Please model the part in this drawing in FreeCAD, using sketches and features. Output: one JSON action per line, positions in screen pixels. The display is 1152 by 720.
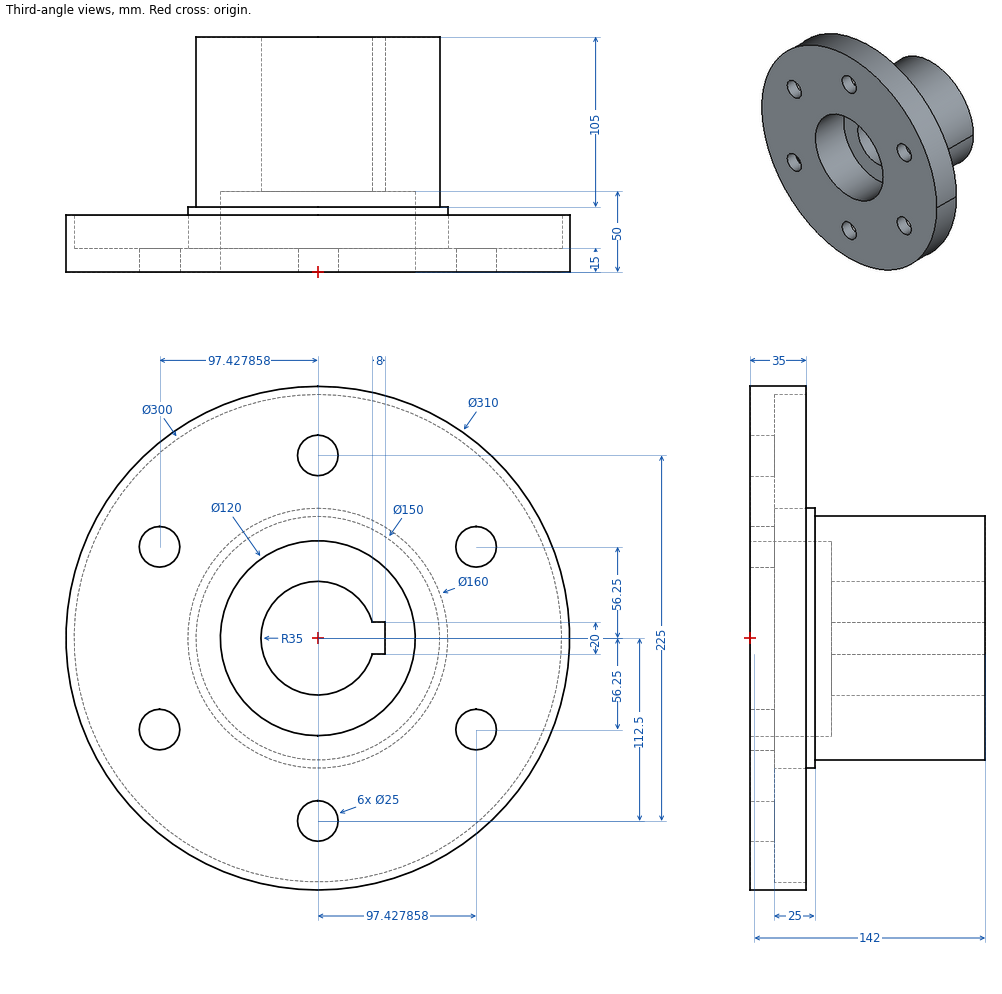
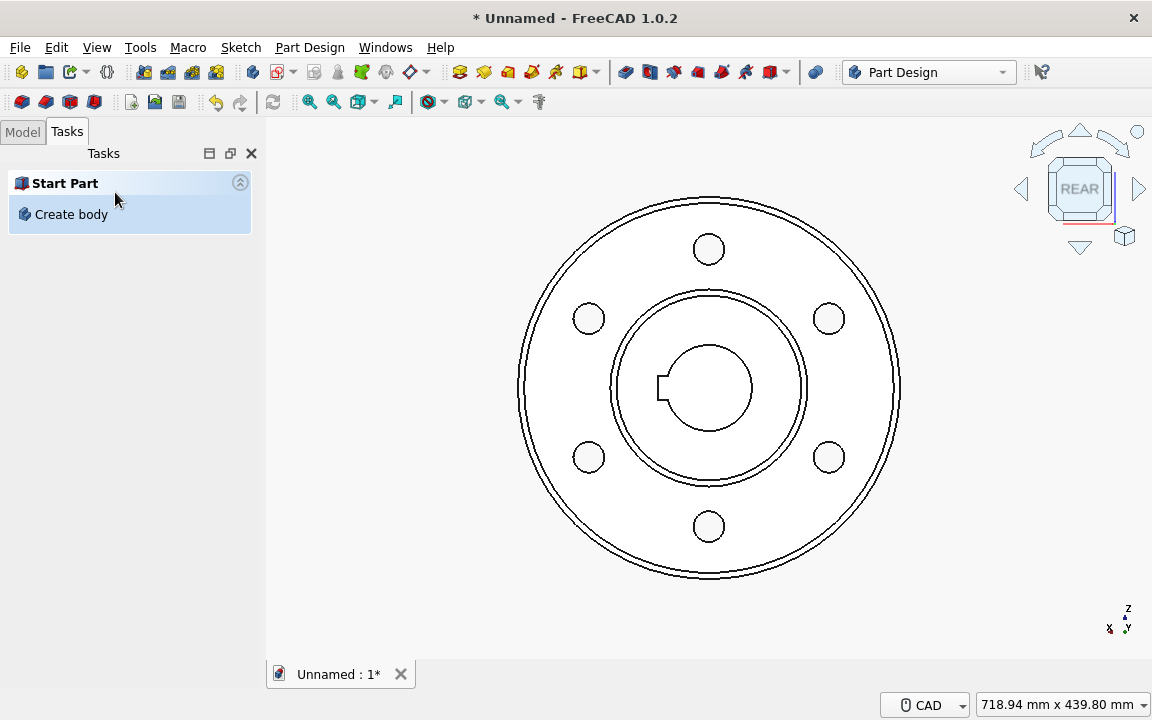
{"action": "key", "text": "0"}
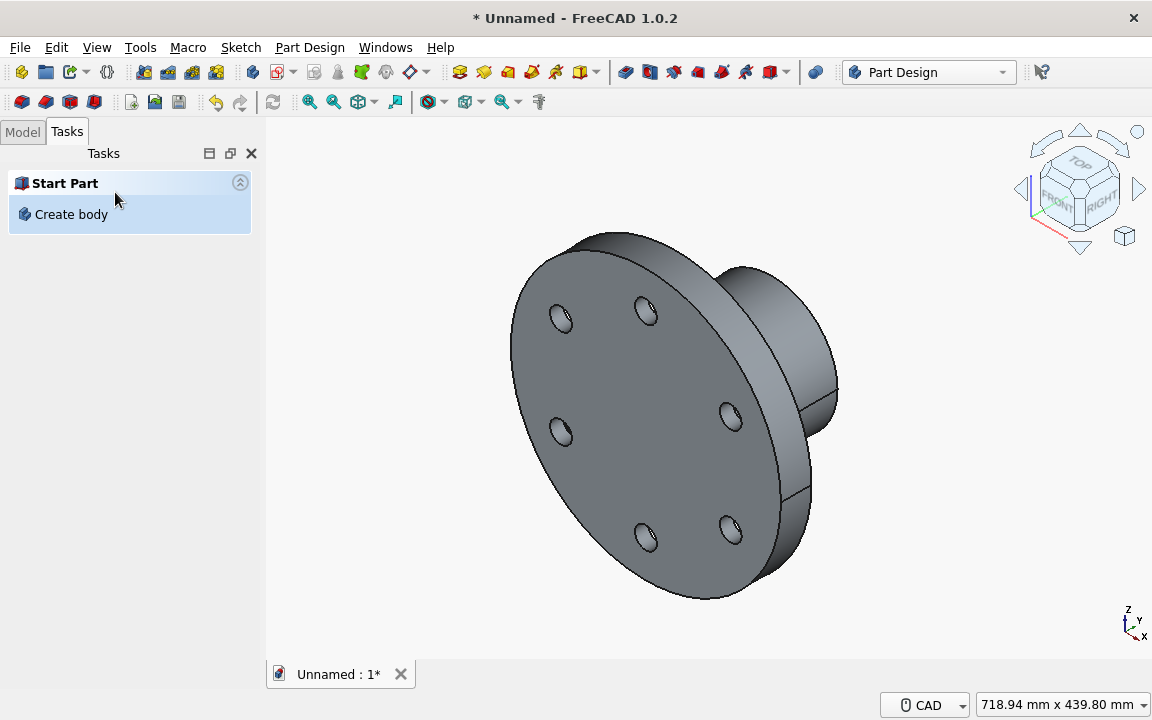
{"action": "left_click", "coordinate": [646, 423]}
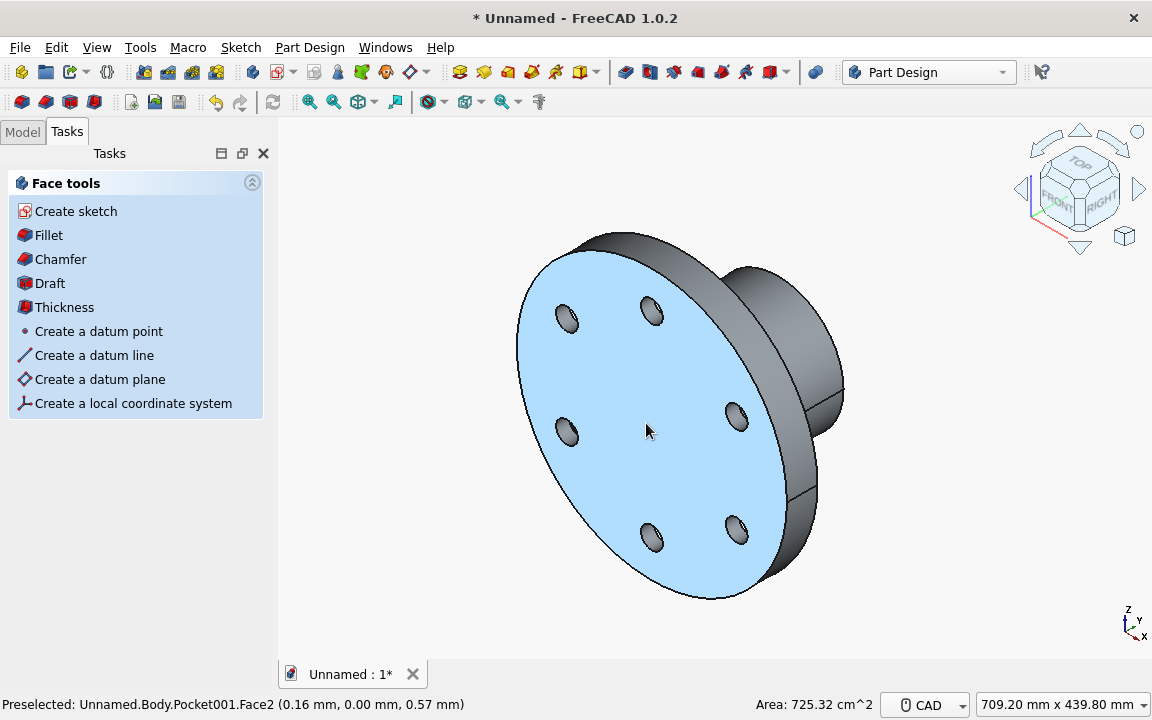
{"action": "left_click", "coordinate": [278, 72]}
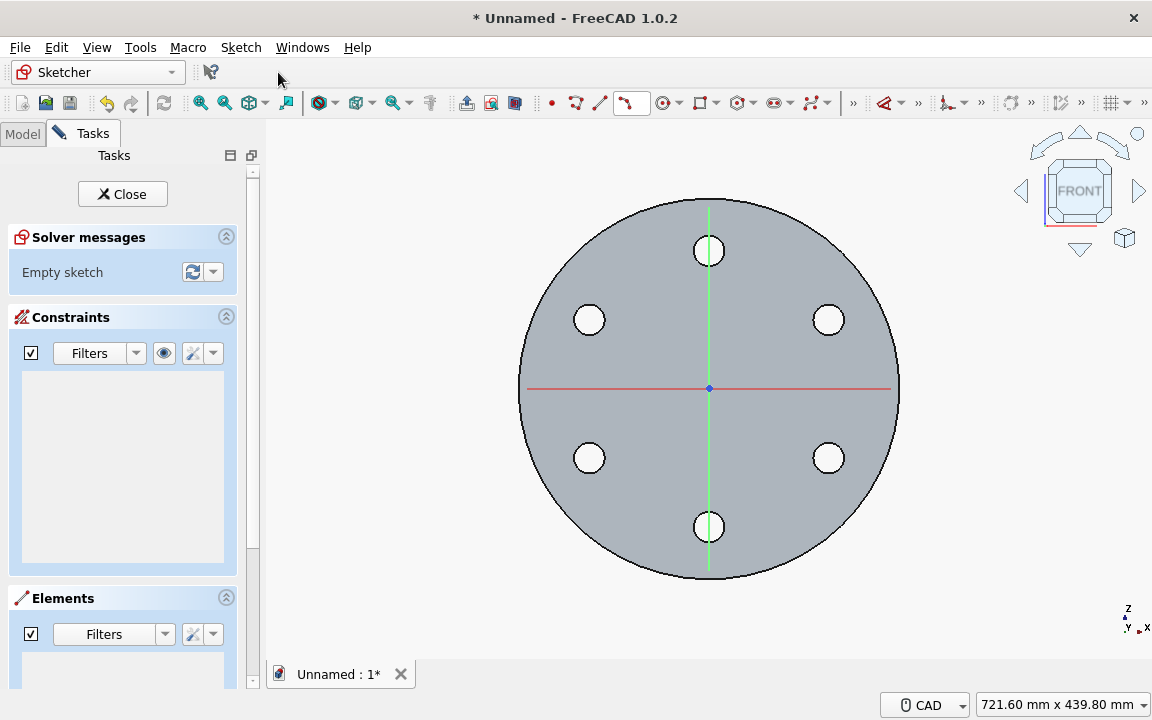
{"action": "scroll", "coordinate": [765, 389], "scroll_direction": "up", "scroll_amount": 4}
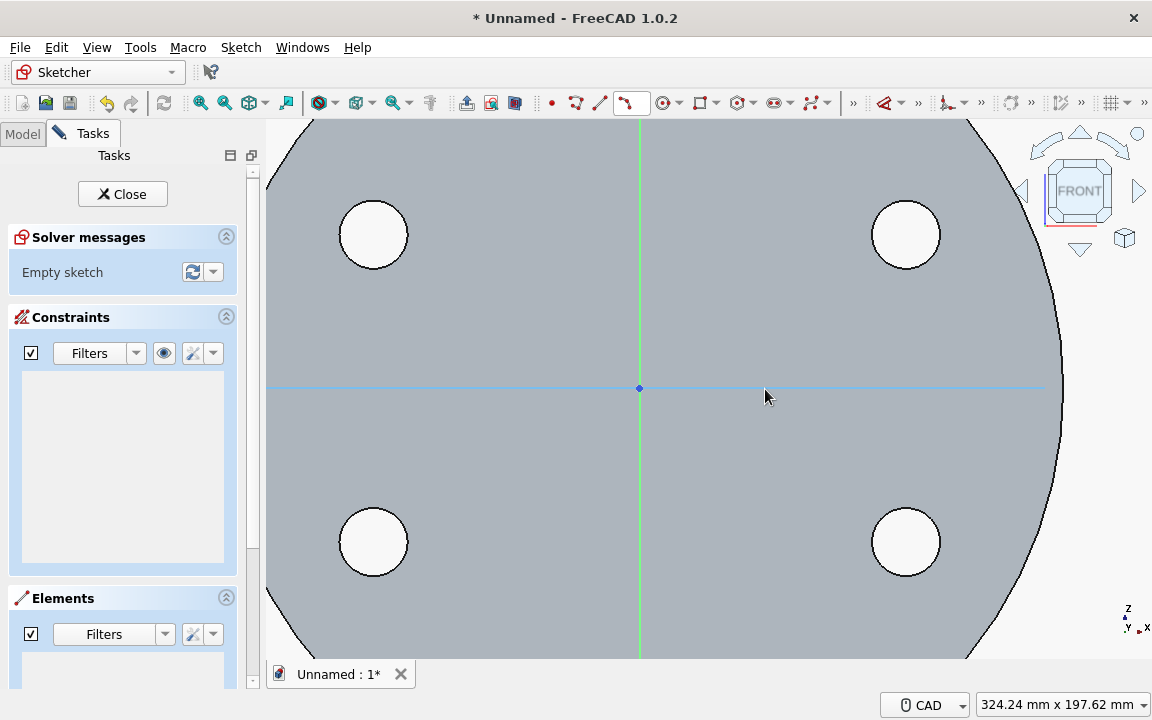
{"action": "left_click", "coordinate": [664, 104]}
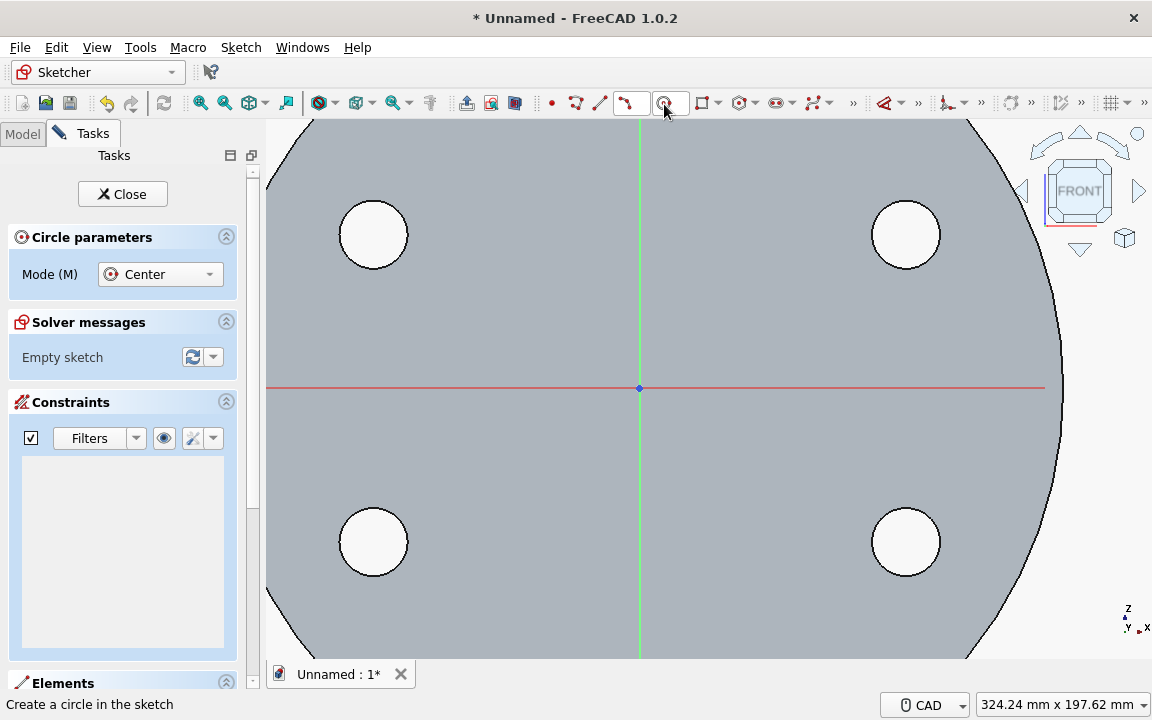
{"action": "left_click", "coordinate": [640, 388]}
{"action": "mouse_move", "coordinate": [756, 272]}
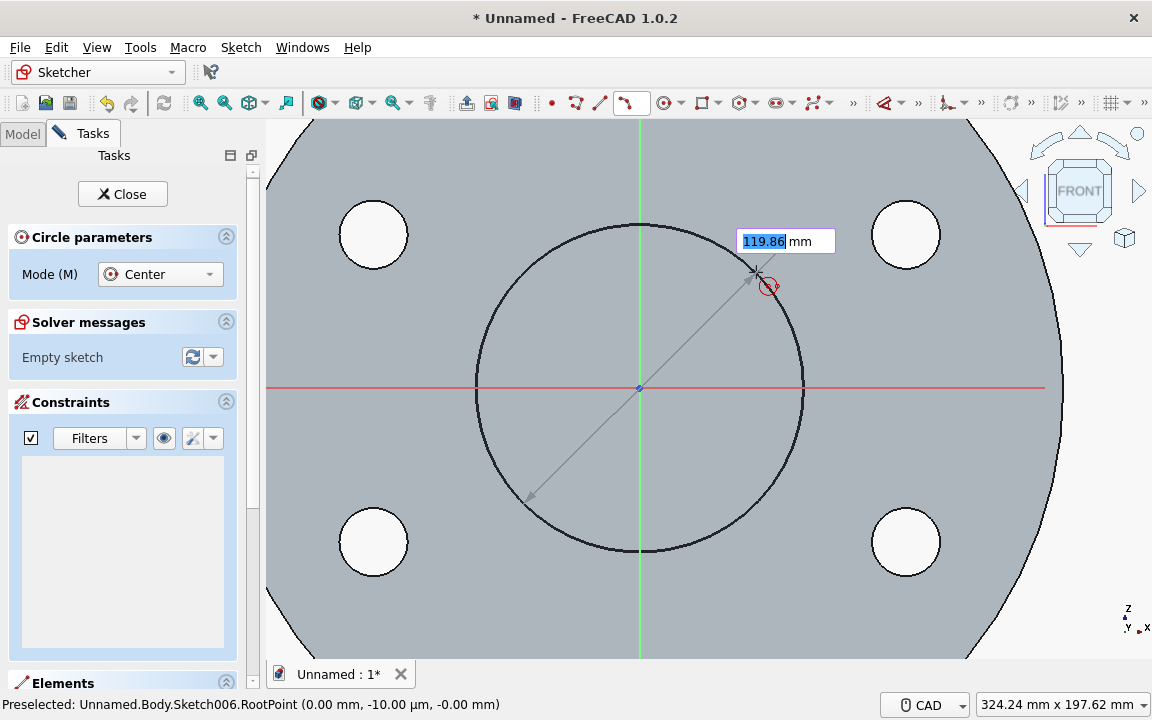
{"action": "type", "text": "120"}
{"action": "key", "text": "Return"}
{"action": "key", "text": "Escape"}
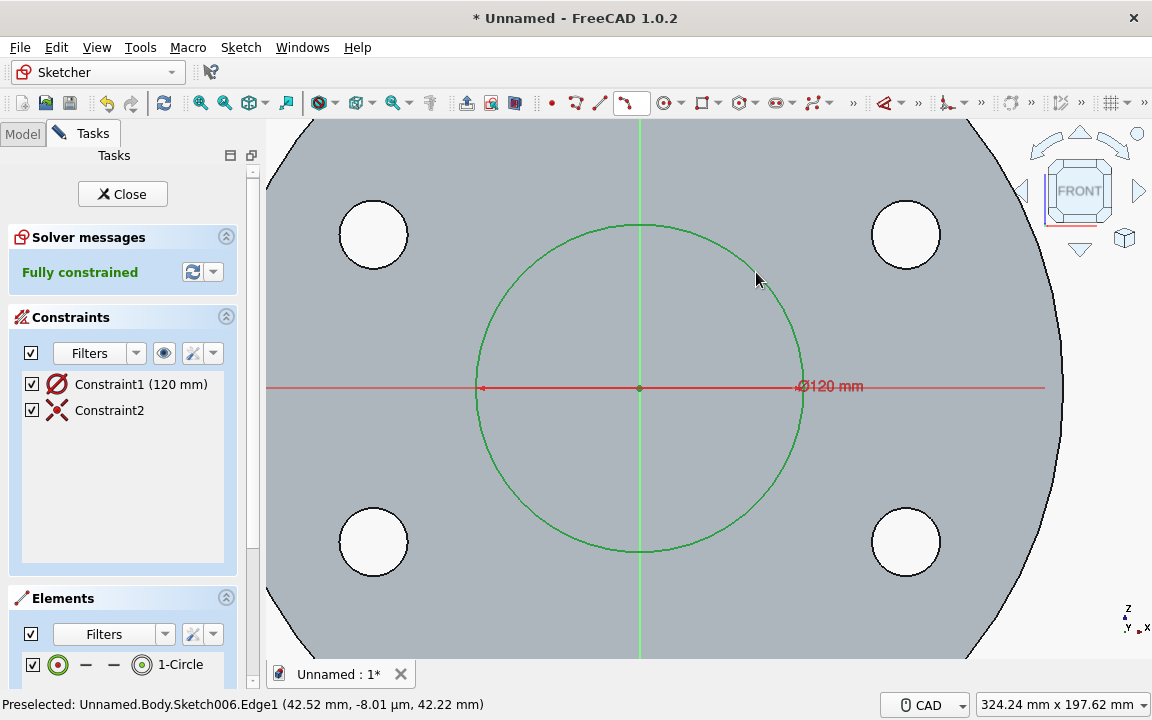
{"action": "left_click", "coordinate": [123, 194]}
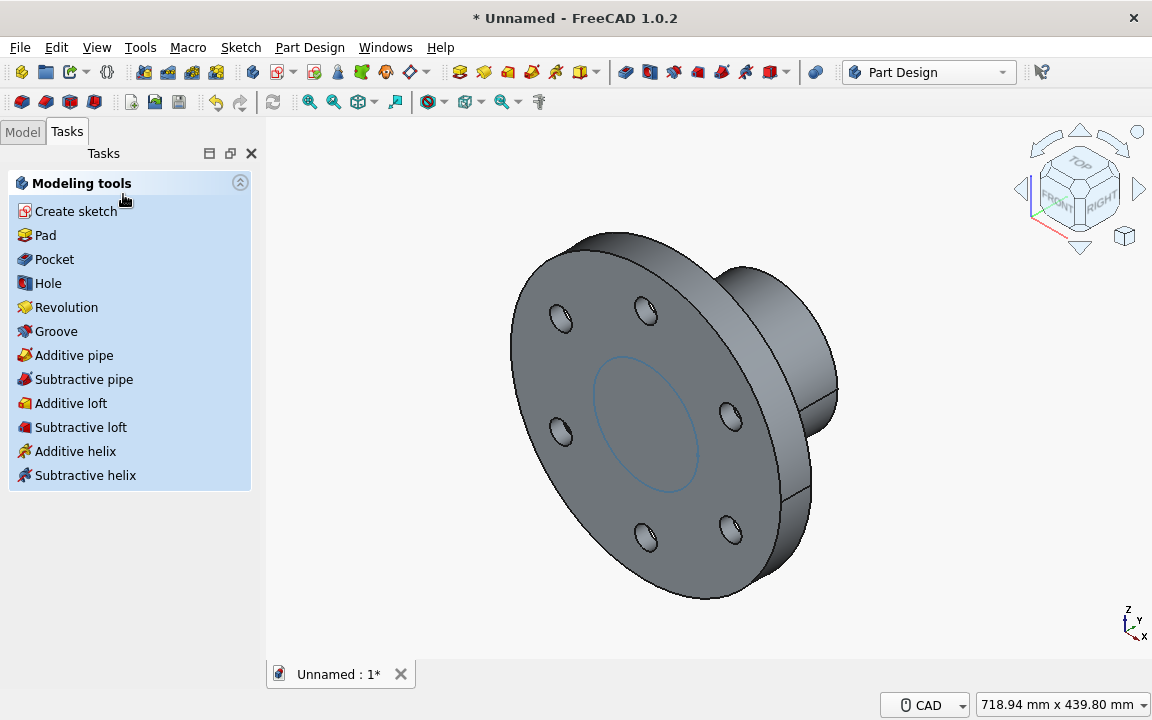
{"action": "left_click", "coordinate": [626, 72]}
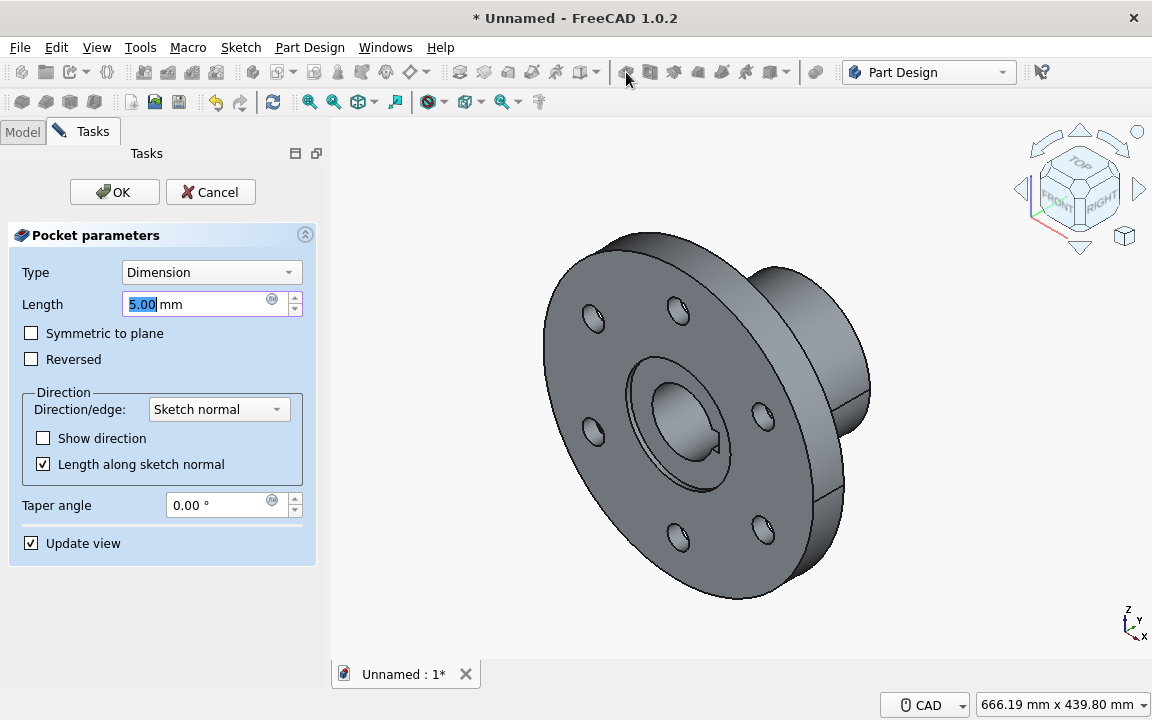
{"action": "type", "text": "50"}
{"action": "key", "text": "Tab"}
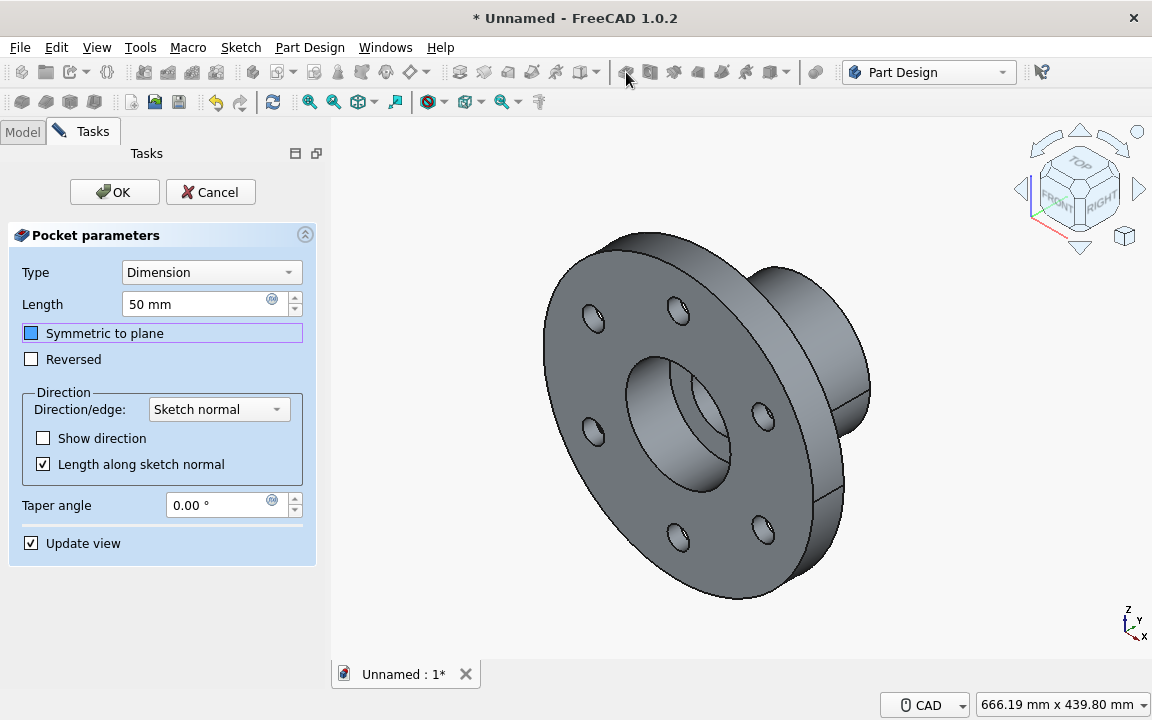
{"action": "left_click", "coordinate": [115, 192]}